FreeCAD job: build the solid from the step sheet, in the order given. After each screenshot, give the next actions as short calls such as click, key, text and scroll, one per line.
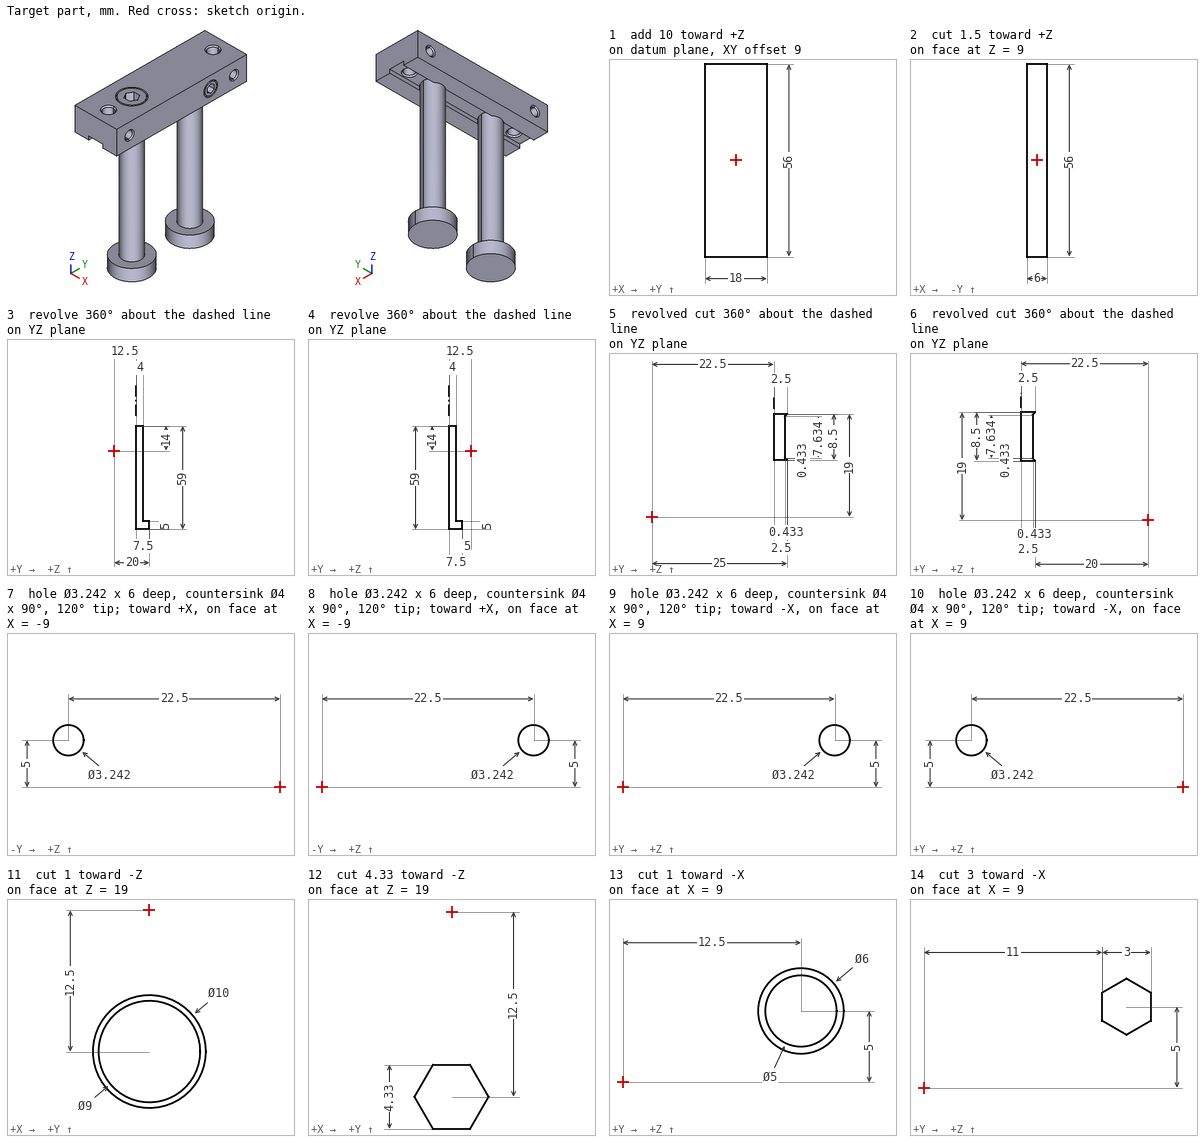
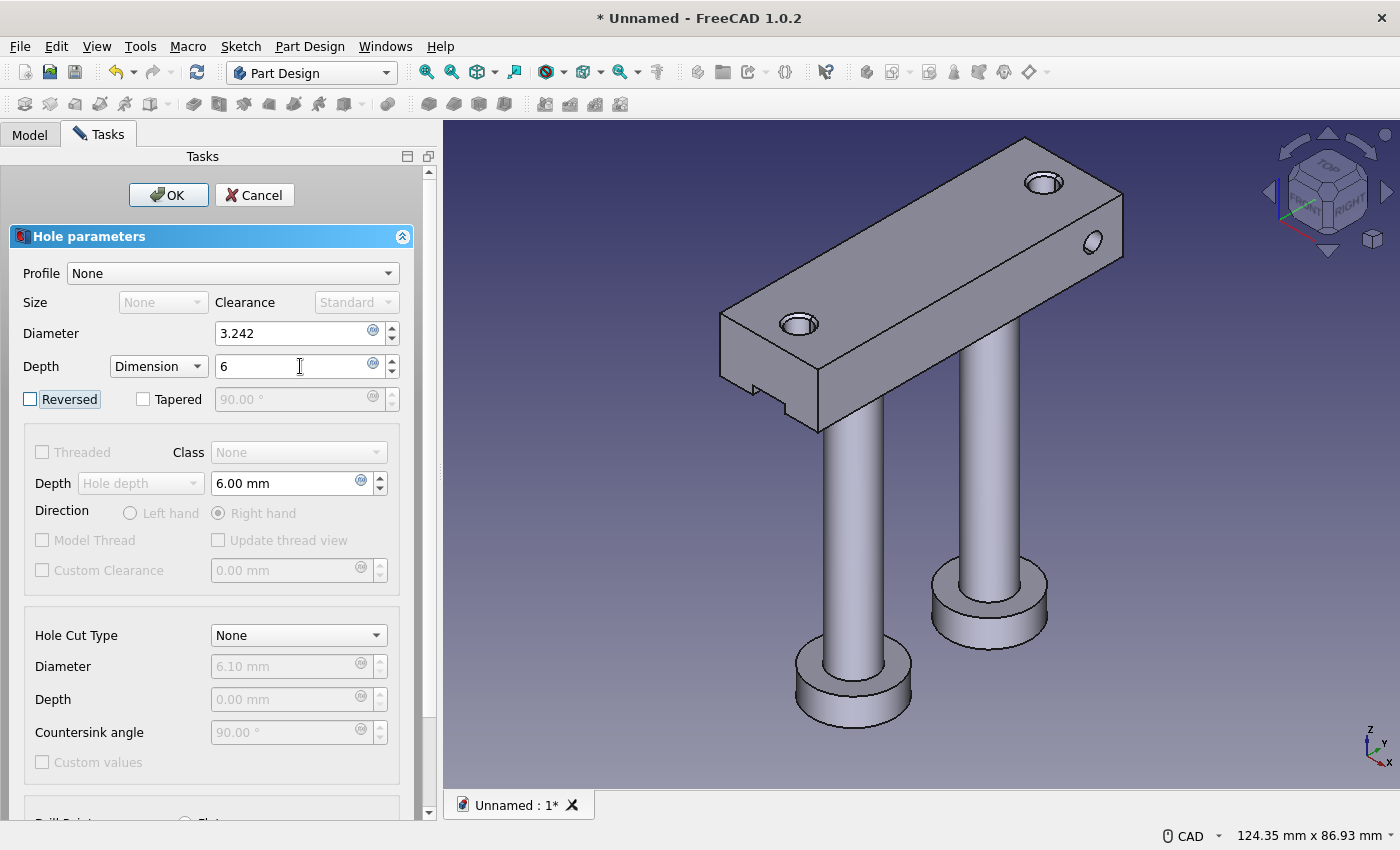
click(300, 636)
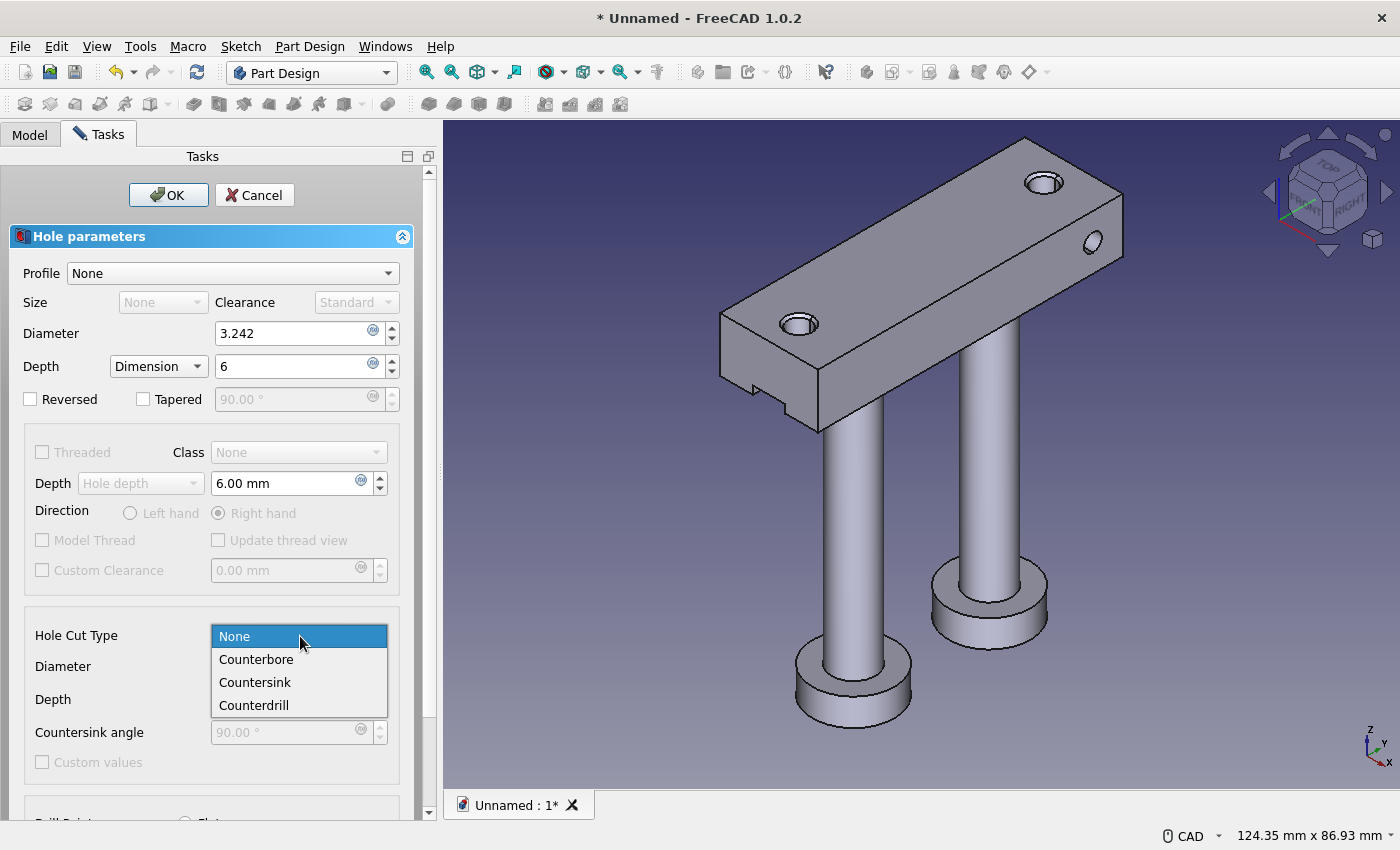
click(298, 682)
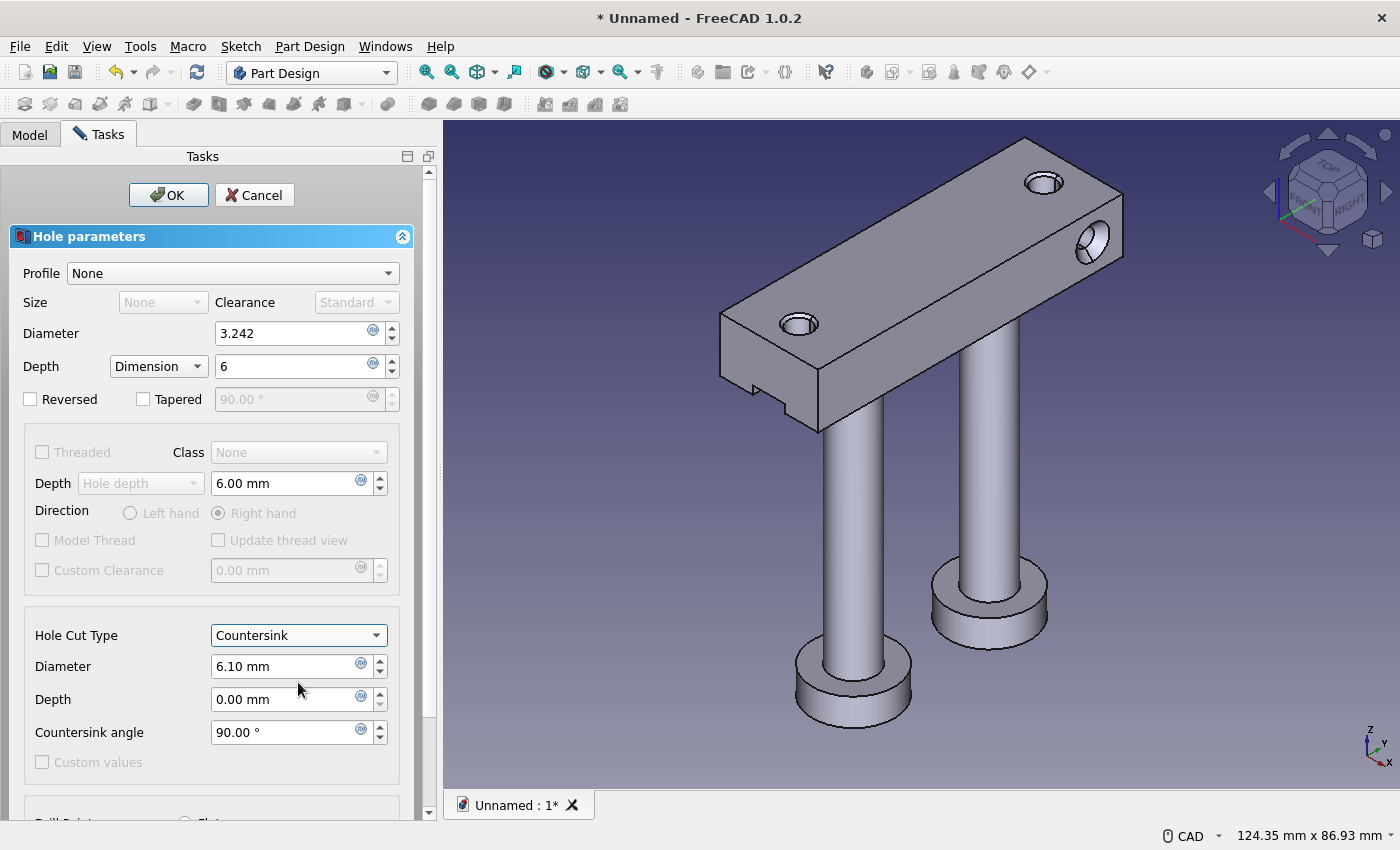
triple_click(292, 666)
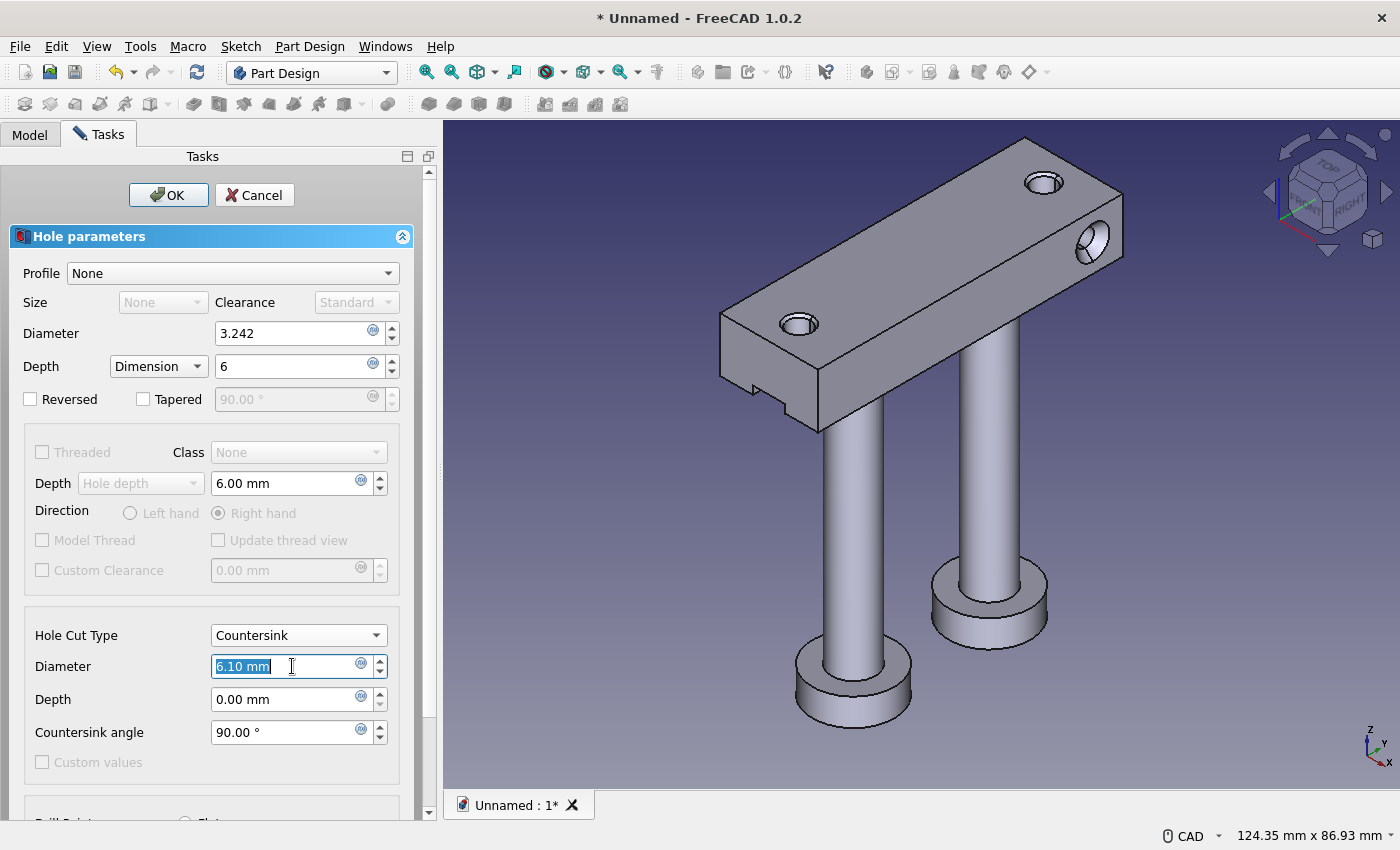
text(4)
key(Tab)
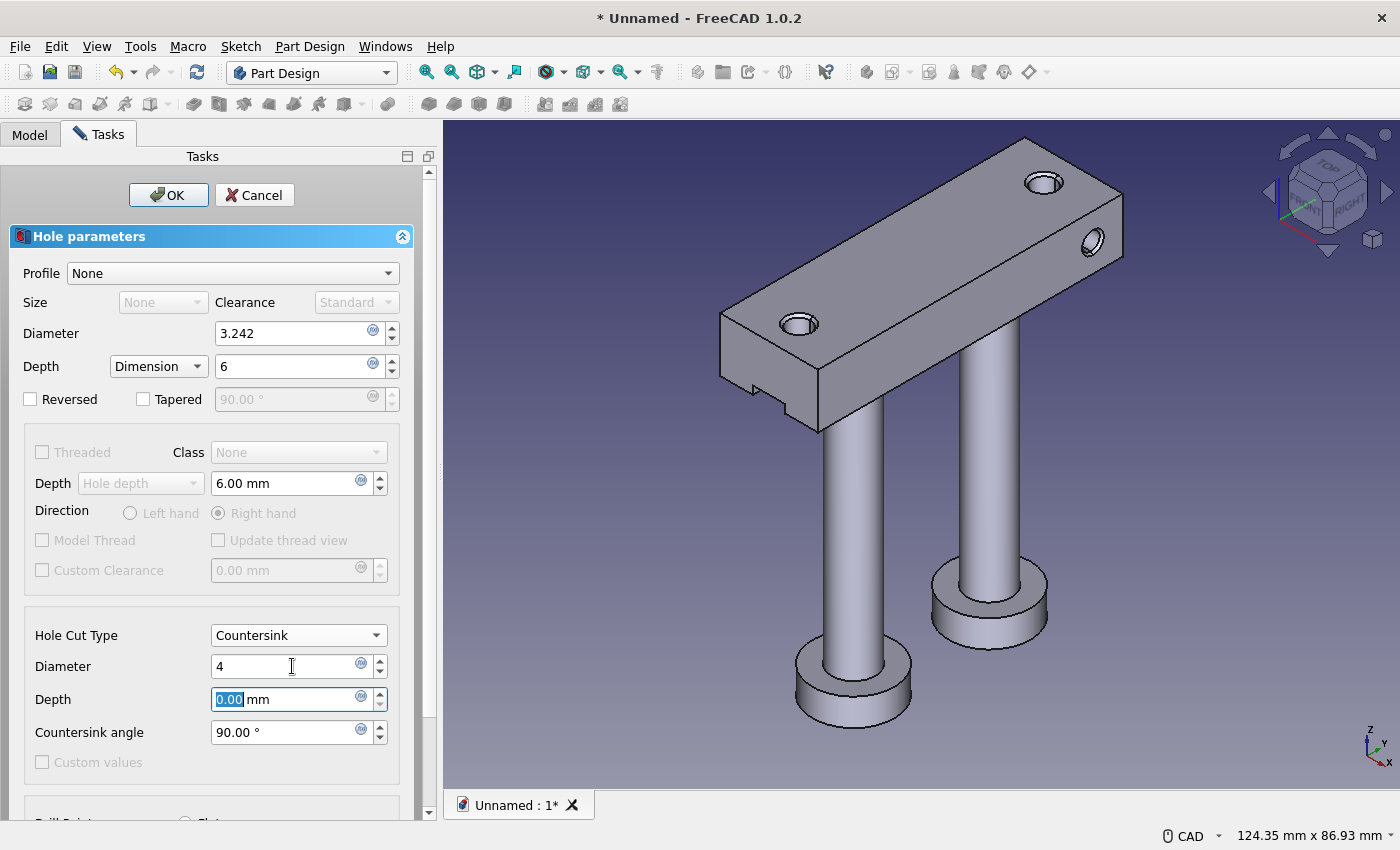
scroll(429, 493, down, 2)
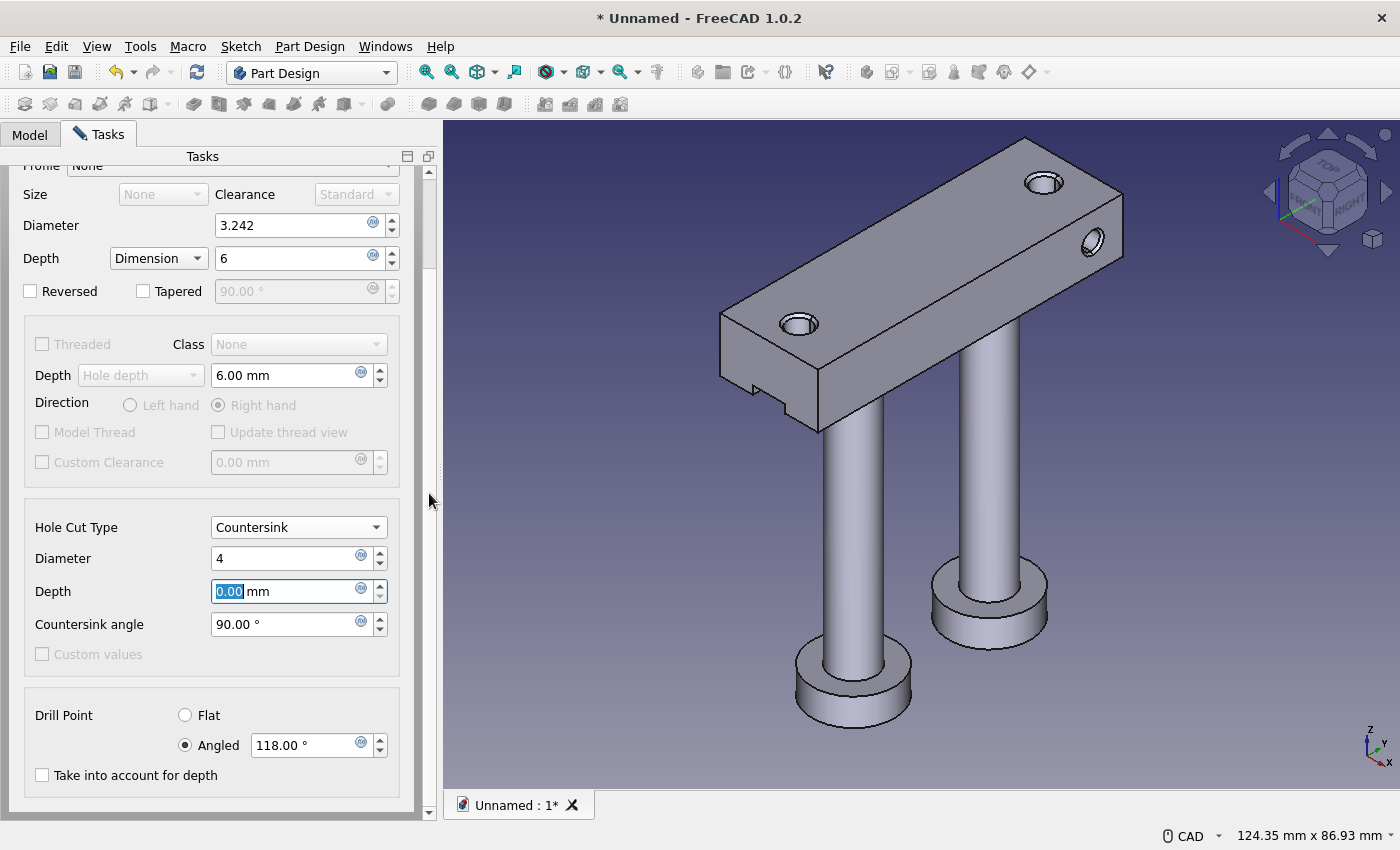
triple_click(312, 746)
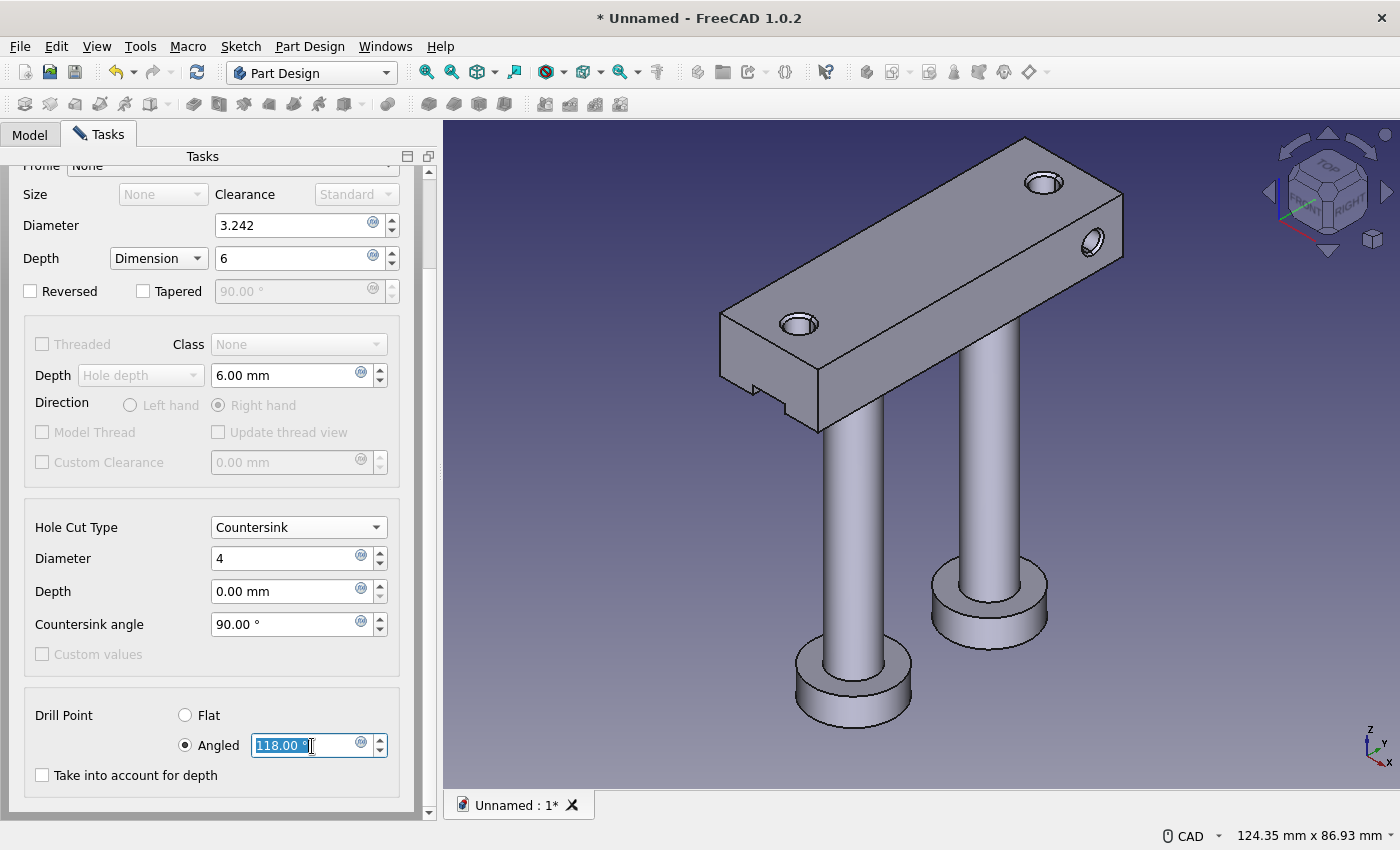
text(120)
key(Tab)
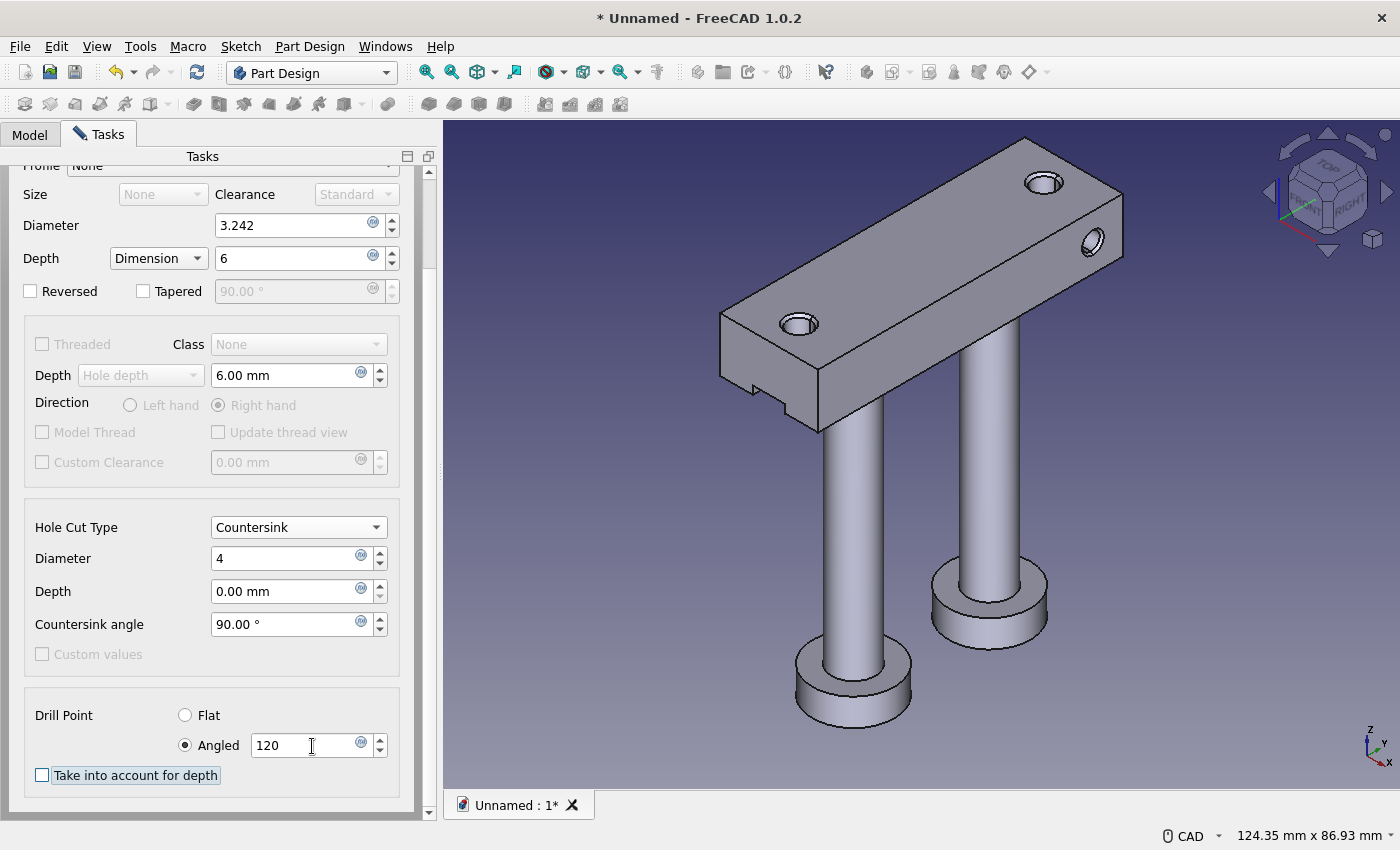
scroll(429, 493, up, 3)